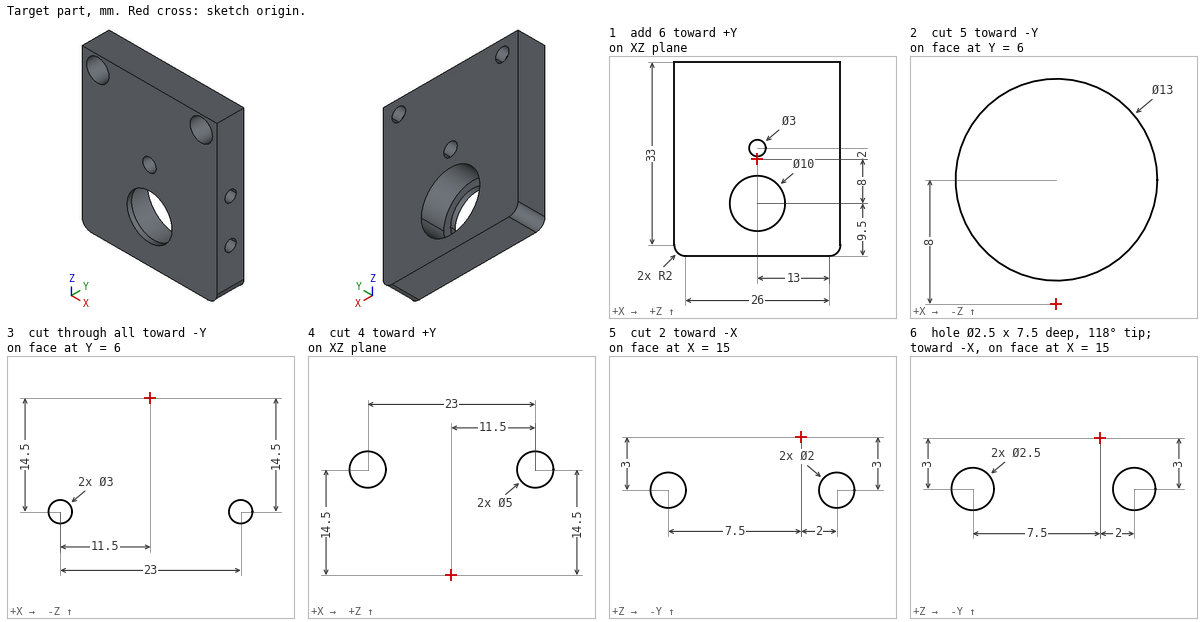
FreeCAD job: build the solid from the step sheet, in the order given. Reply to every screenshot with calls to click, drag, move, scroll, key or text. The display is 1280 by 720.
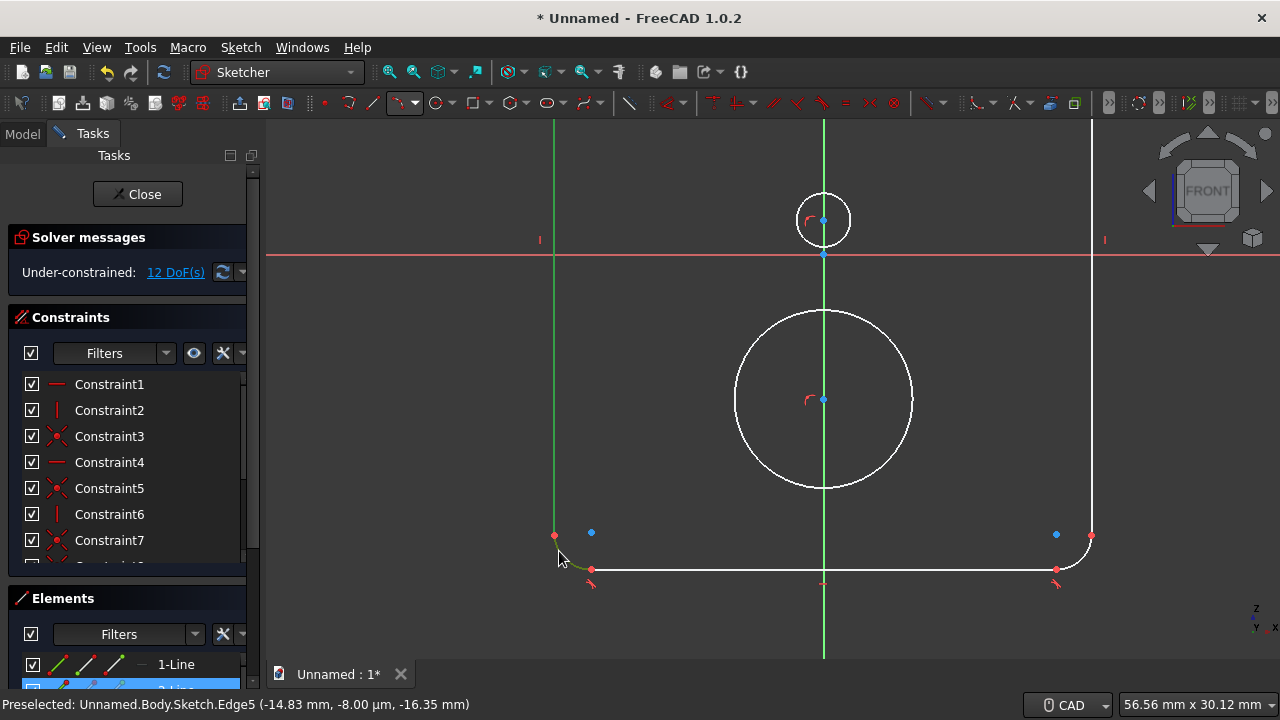
click(822, 104)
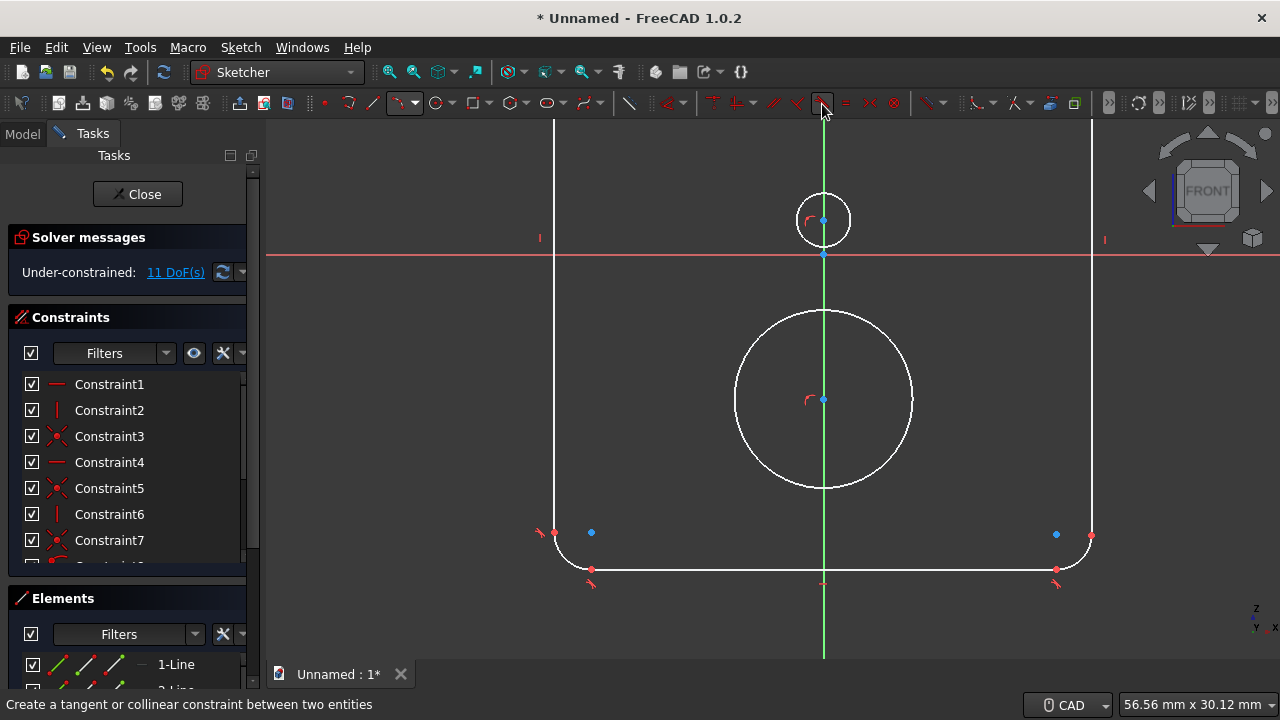
click(1092, 358)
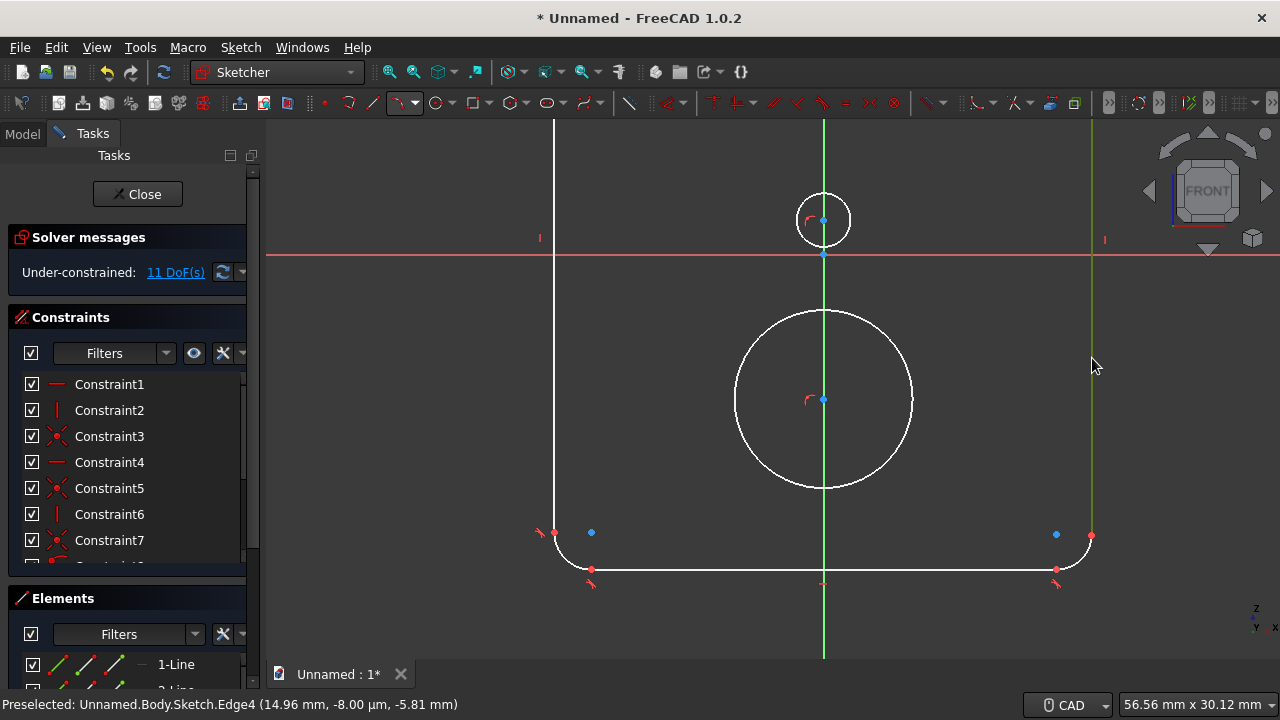
click(1072, 566)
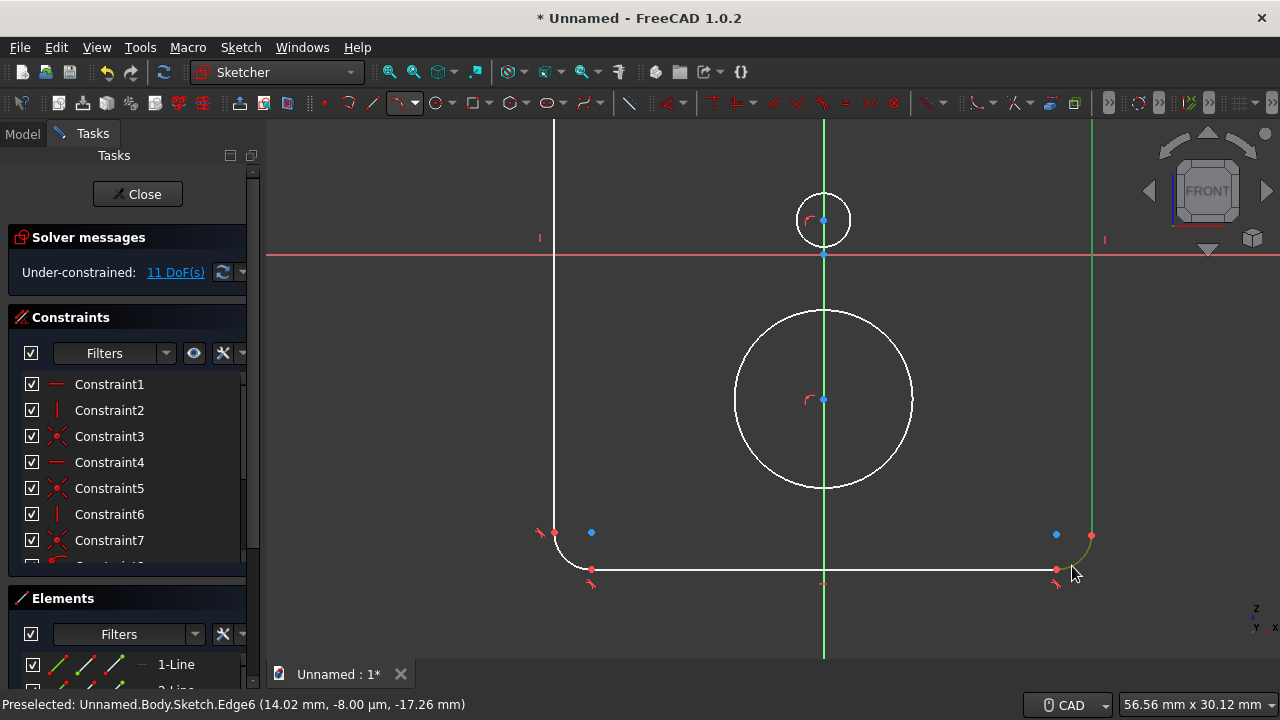
key(t)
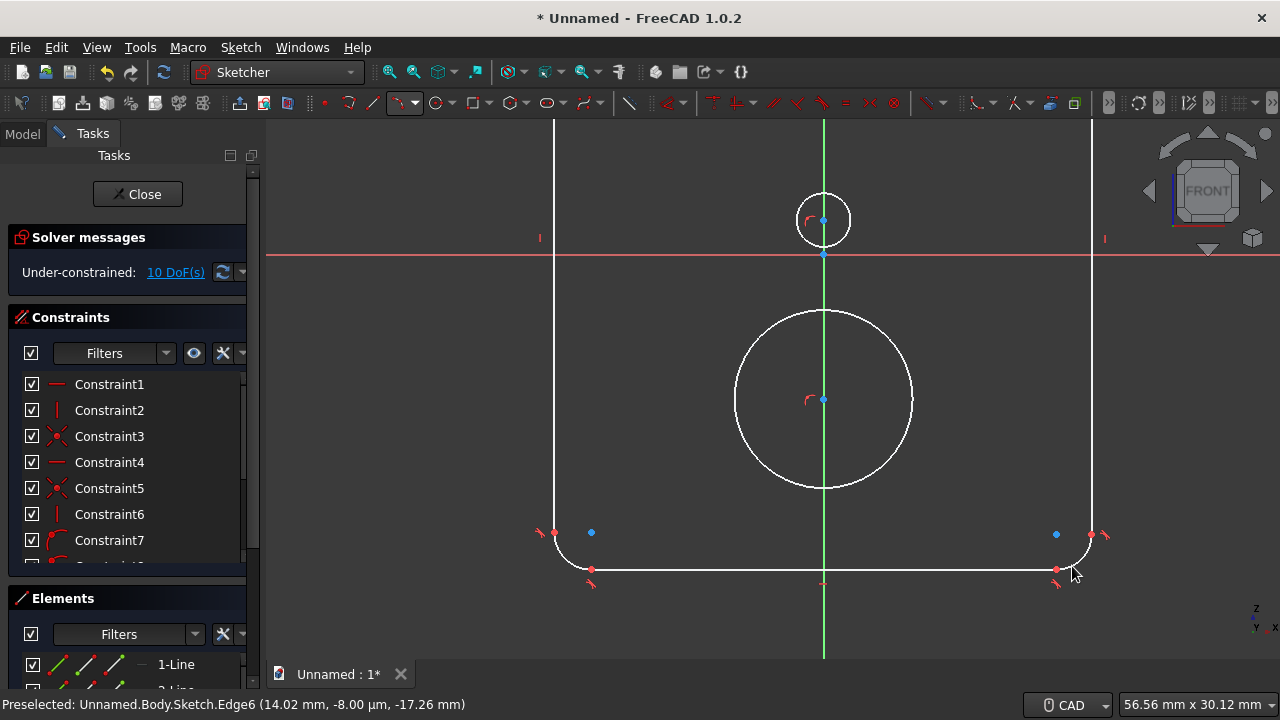
click(558, 549)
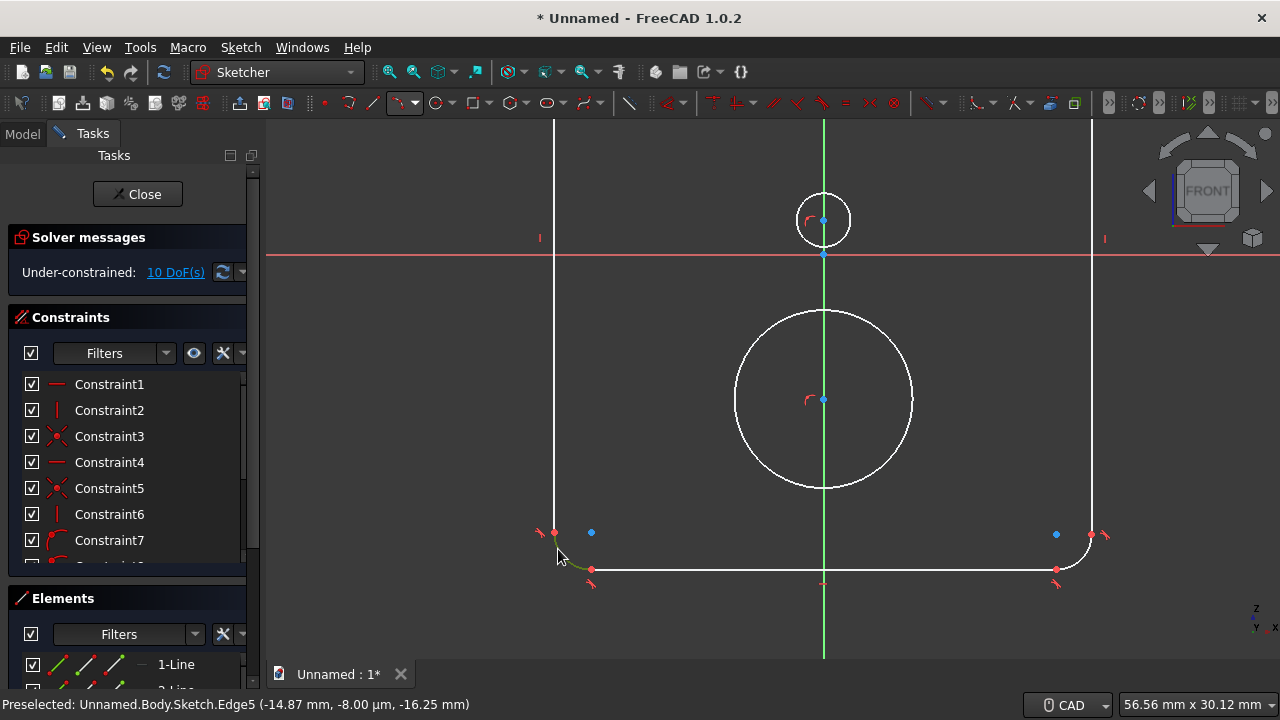
click(1072, 566)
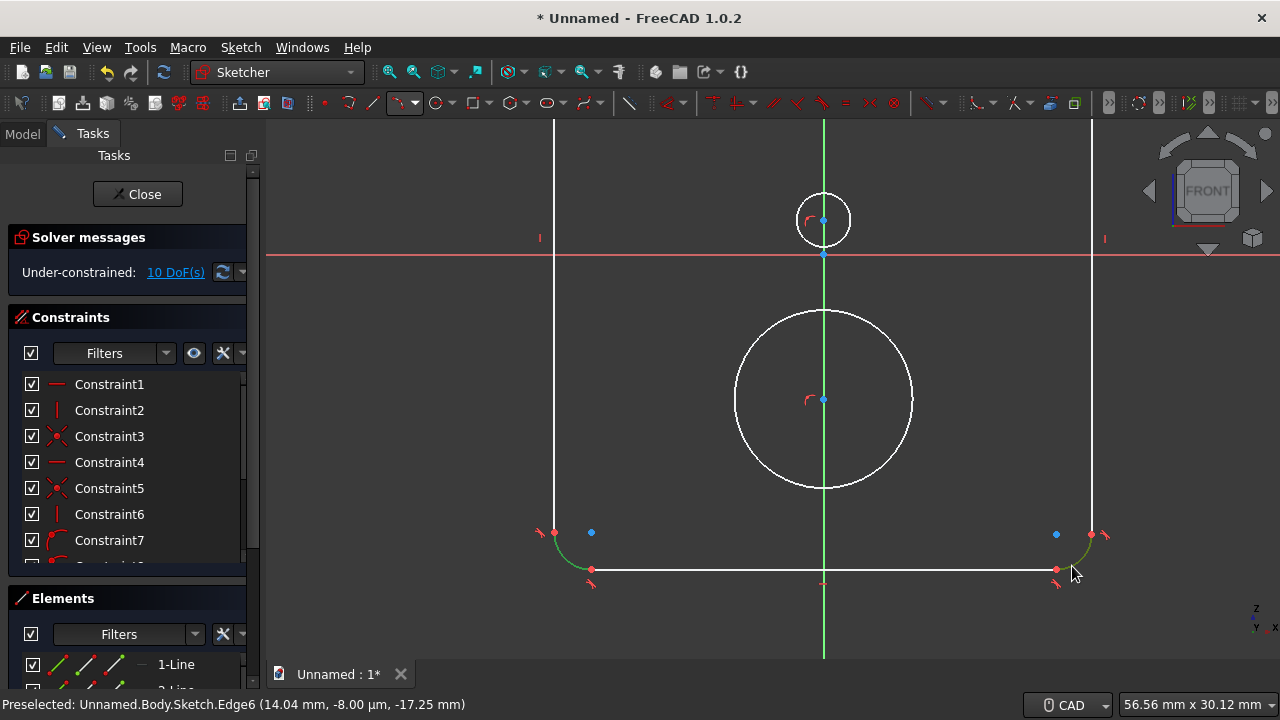
key(e)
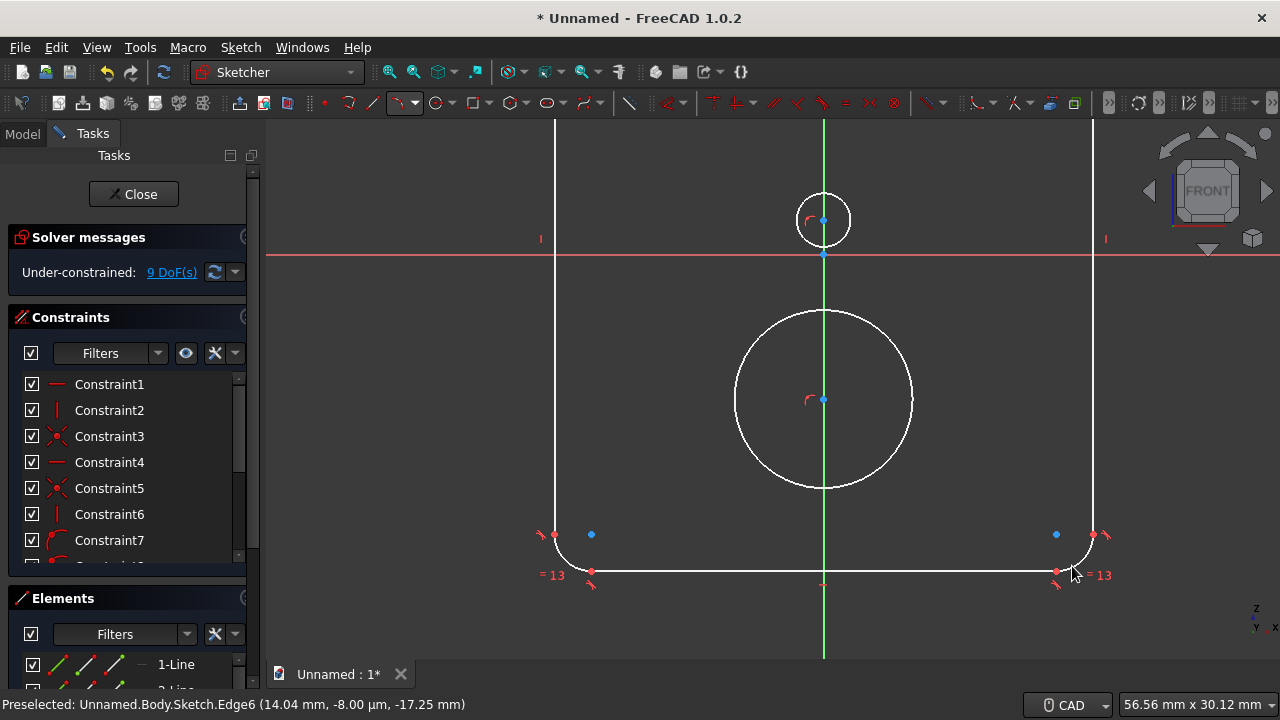
key(d)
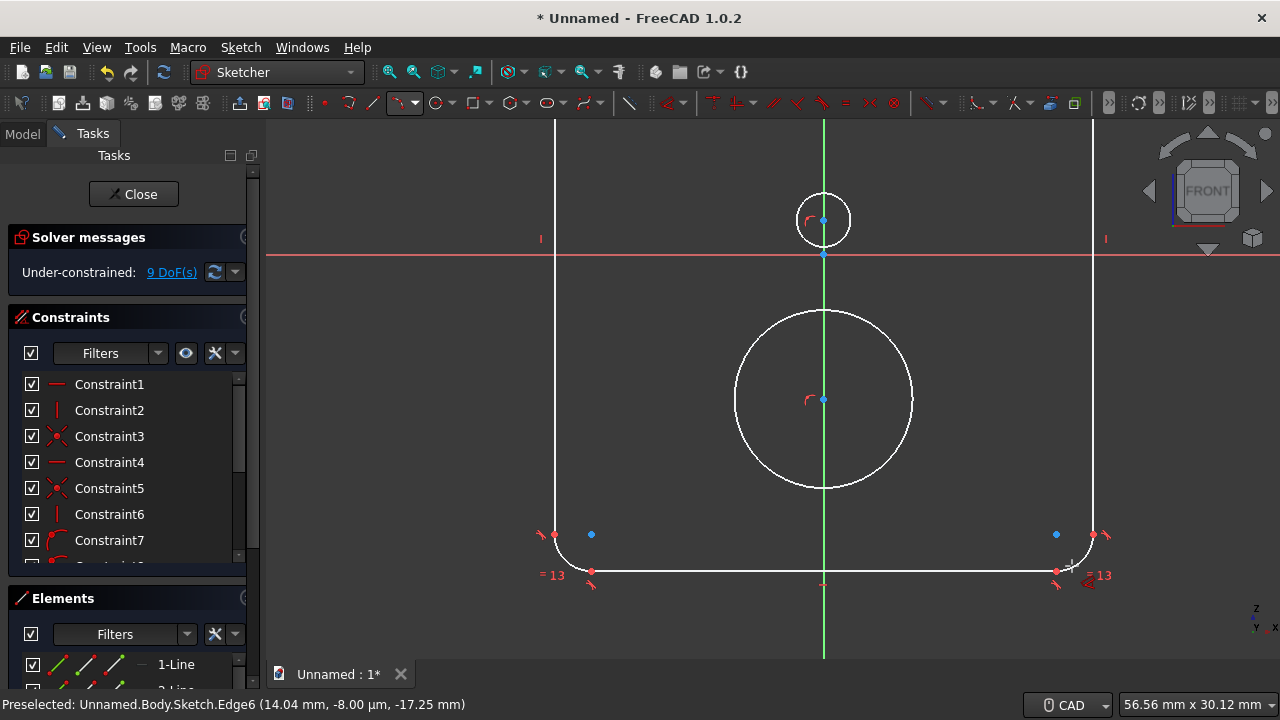
click(559, 551)
click(531, 566)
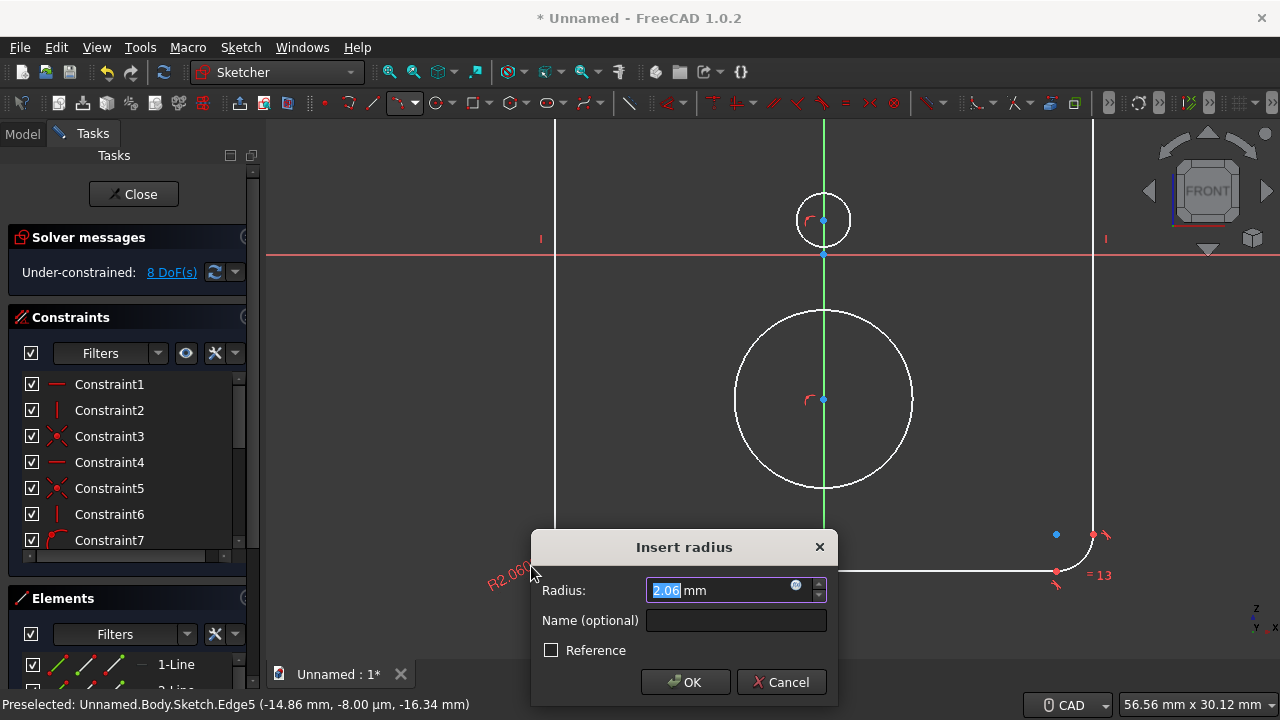
text(2)
key(Return)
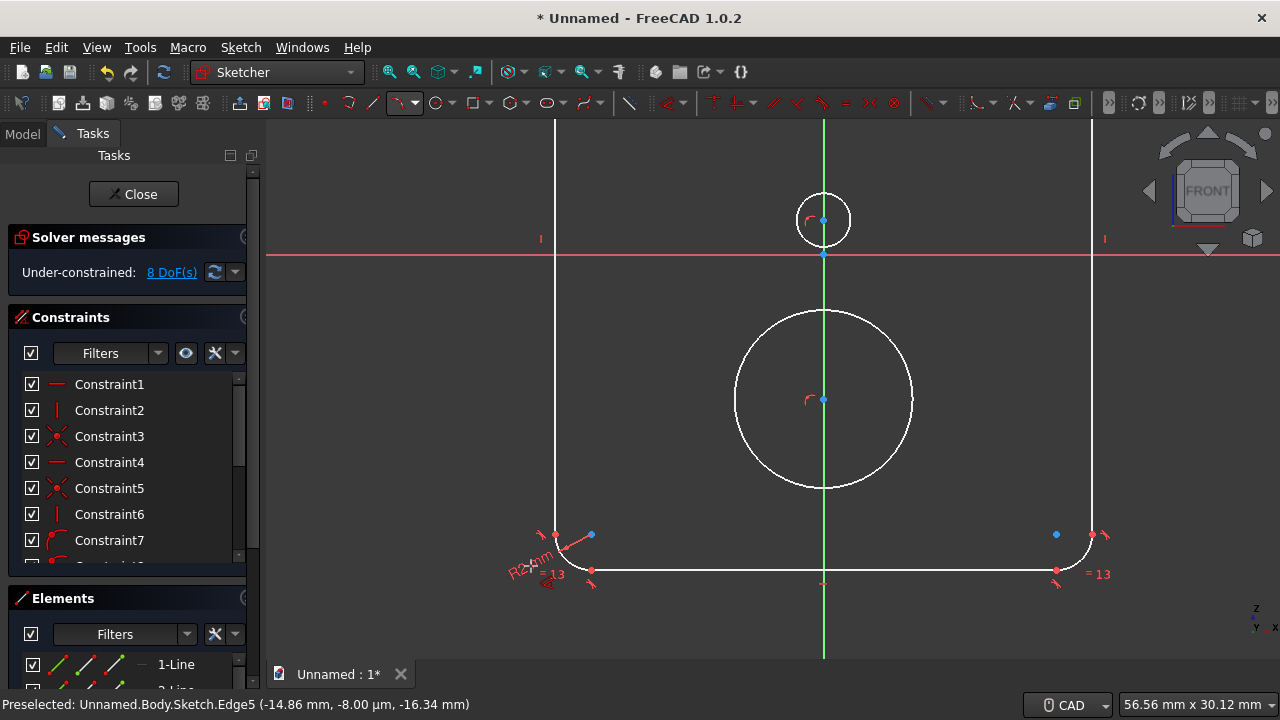
click(842, 201)
click(864, 178)